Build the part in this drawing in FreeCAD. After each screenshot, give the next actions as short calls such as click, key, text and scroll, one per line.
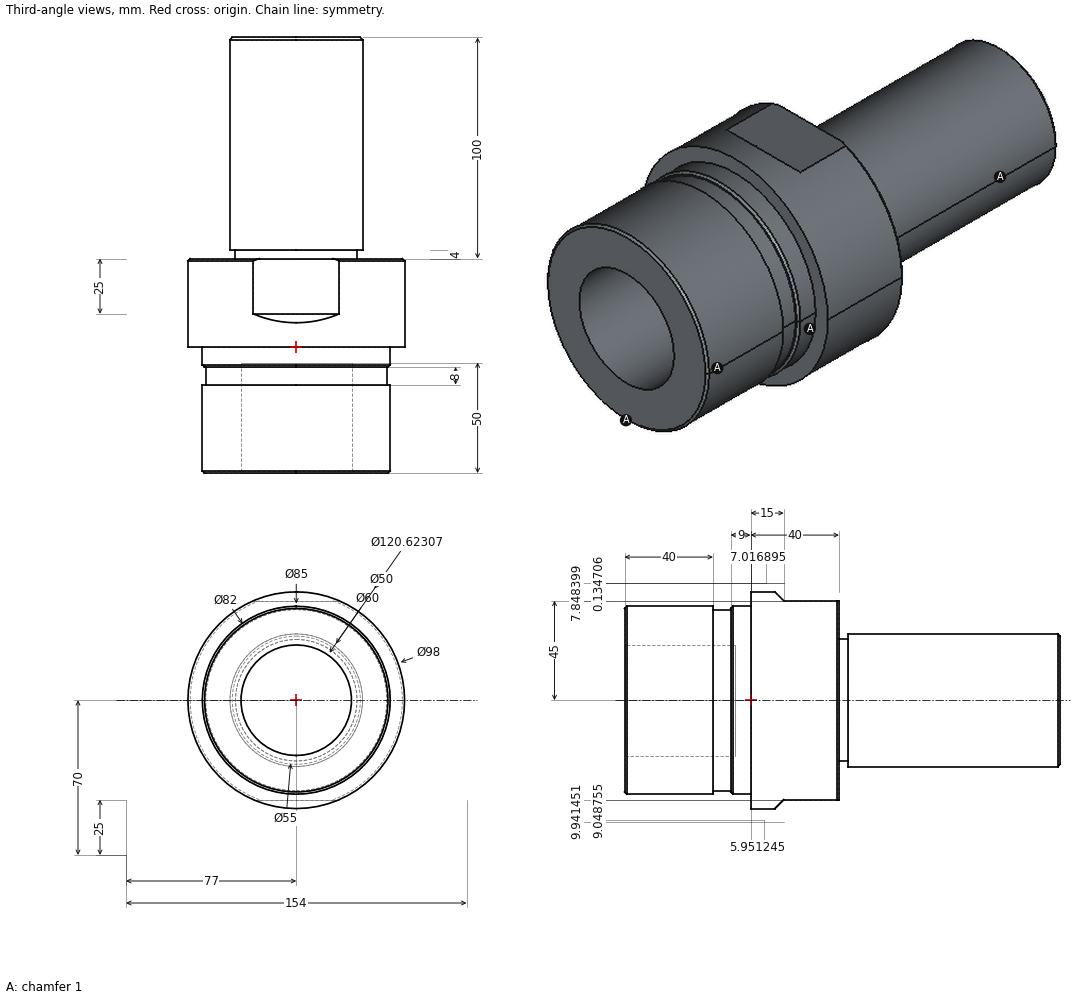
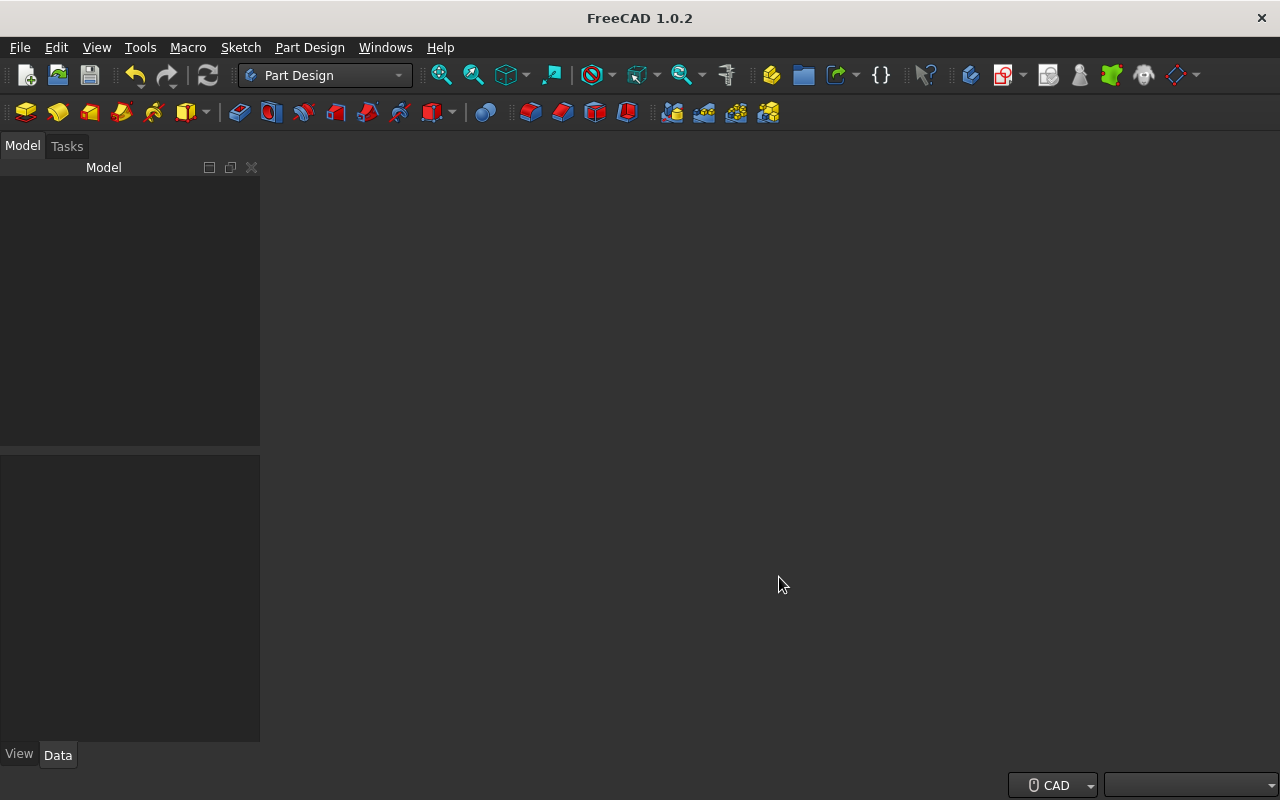
click(26, 76)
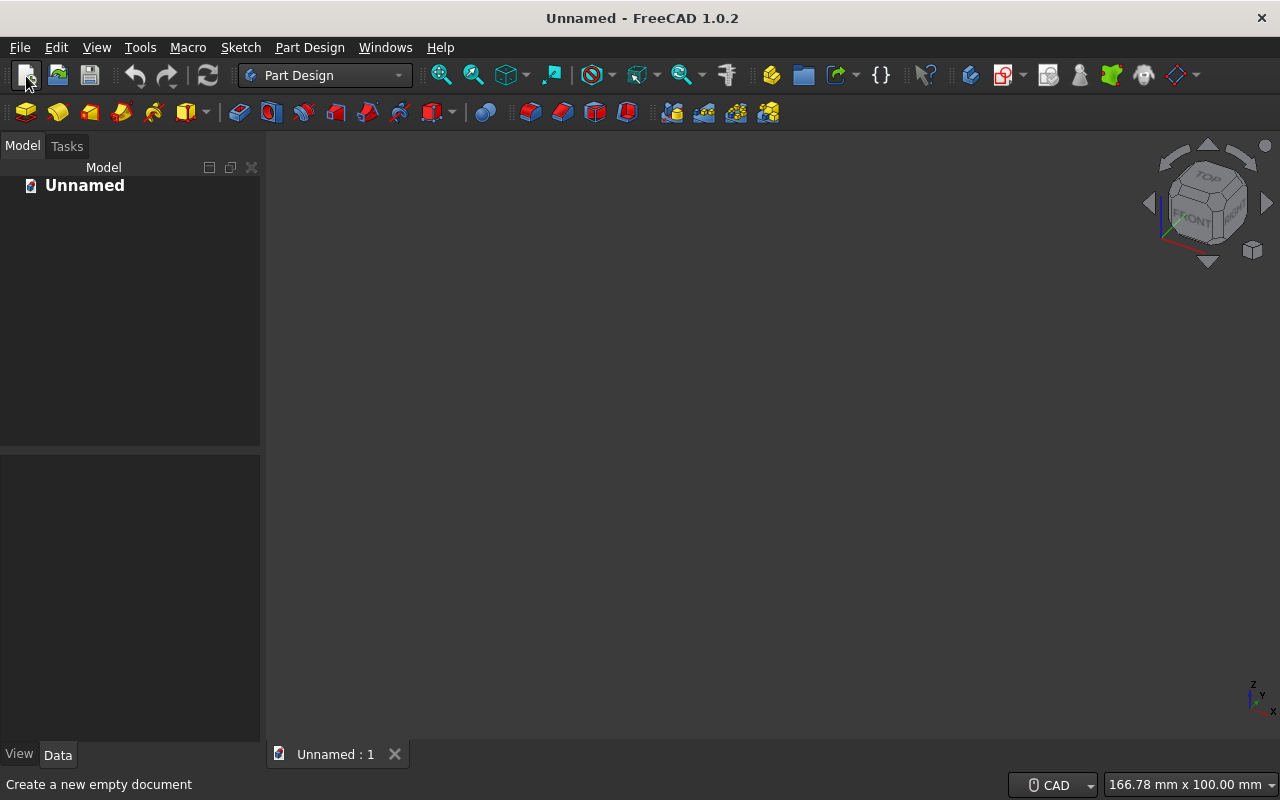
click(1004, 76)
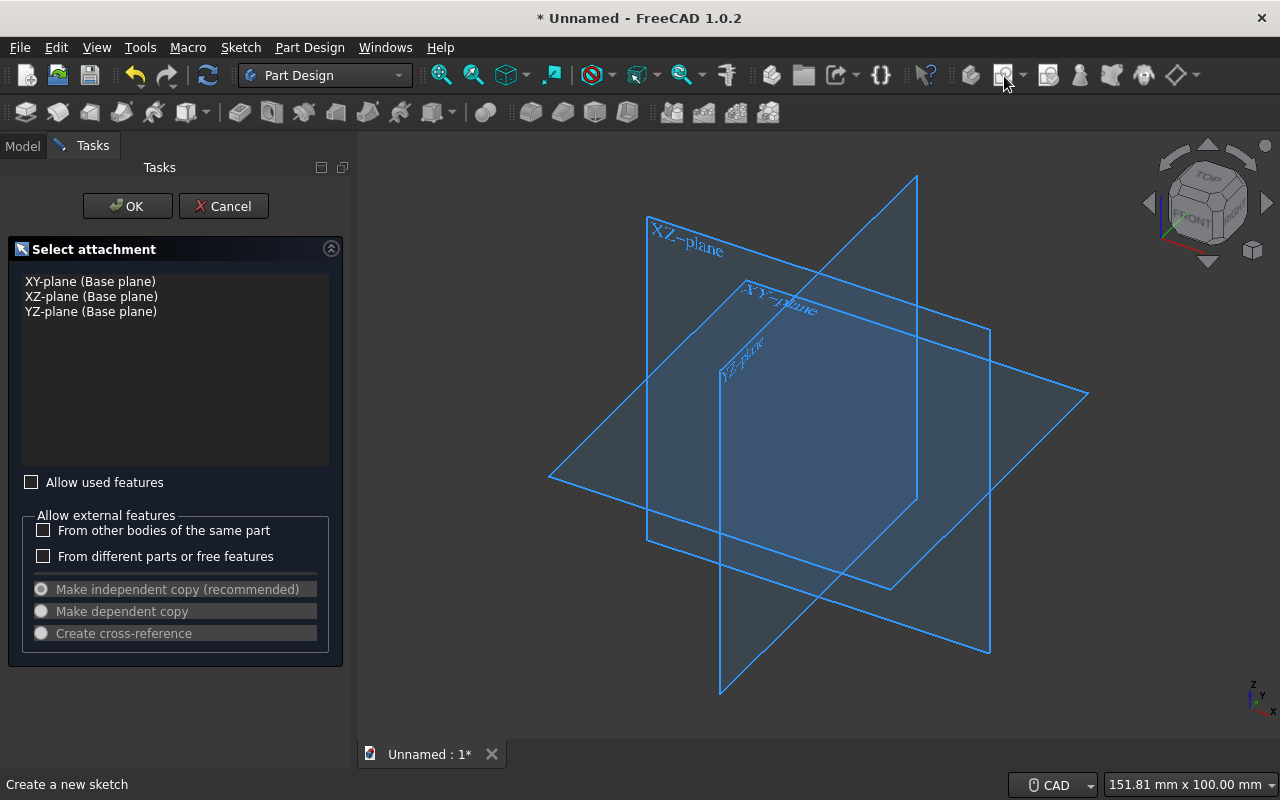
click(82, 296)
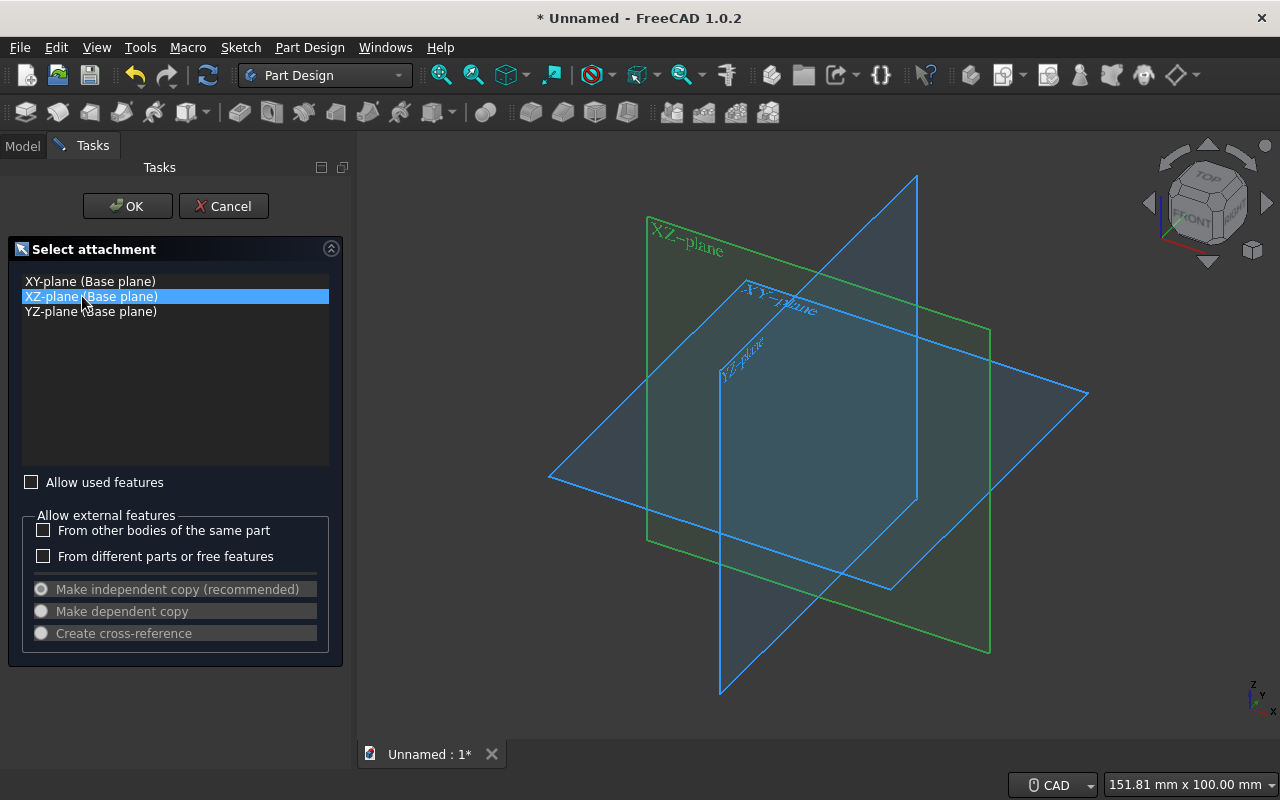
click(128, 206)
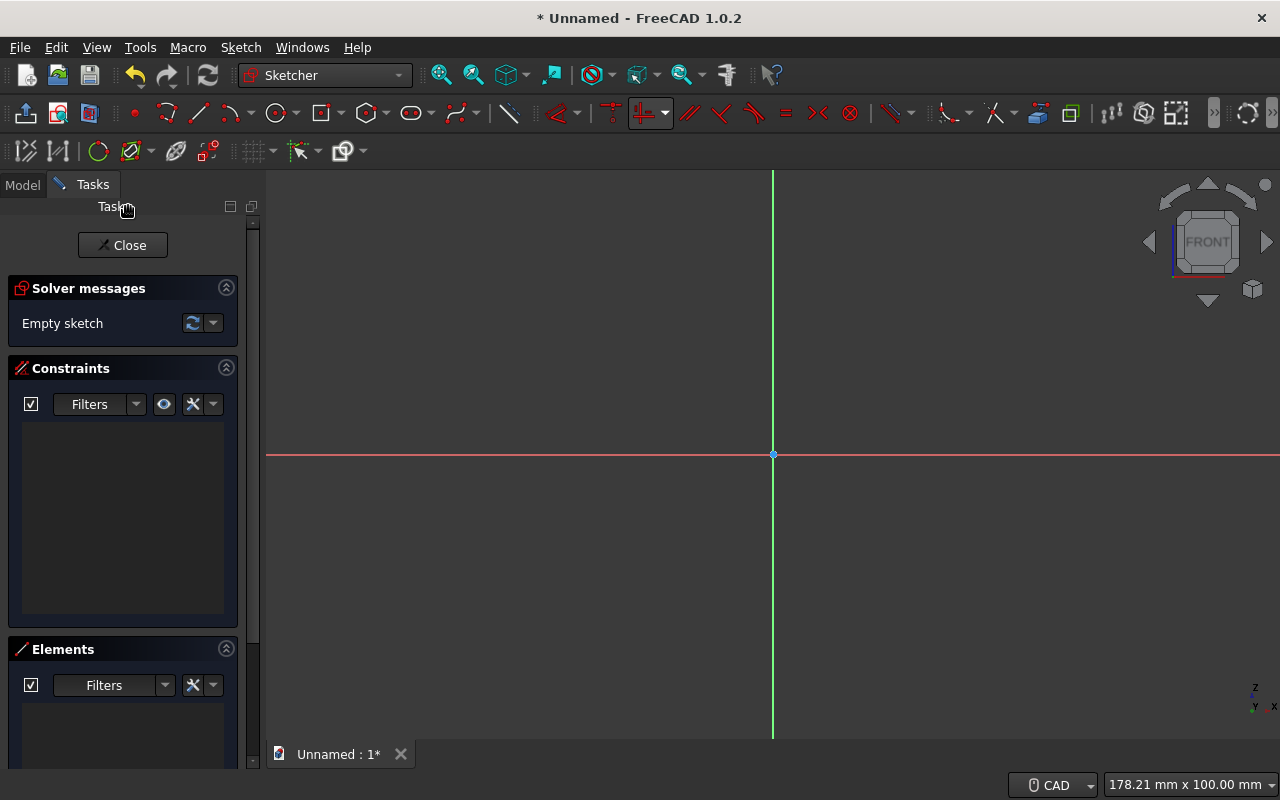
scroll(565, 455, down, 2)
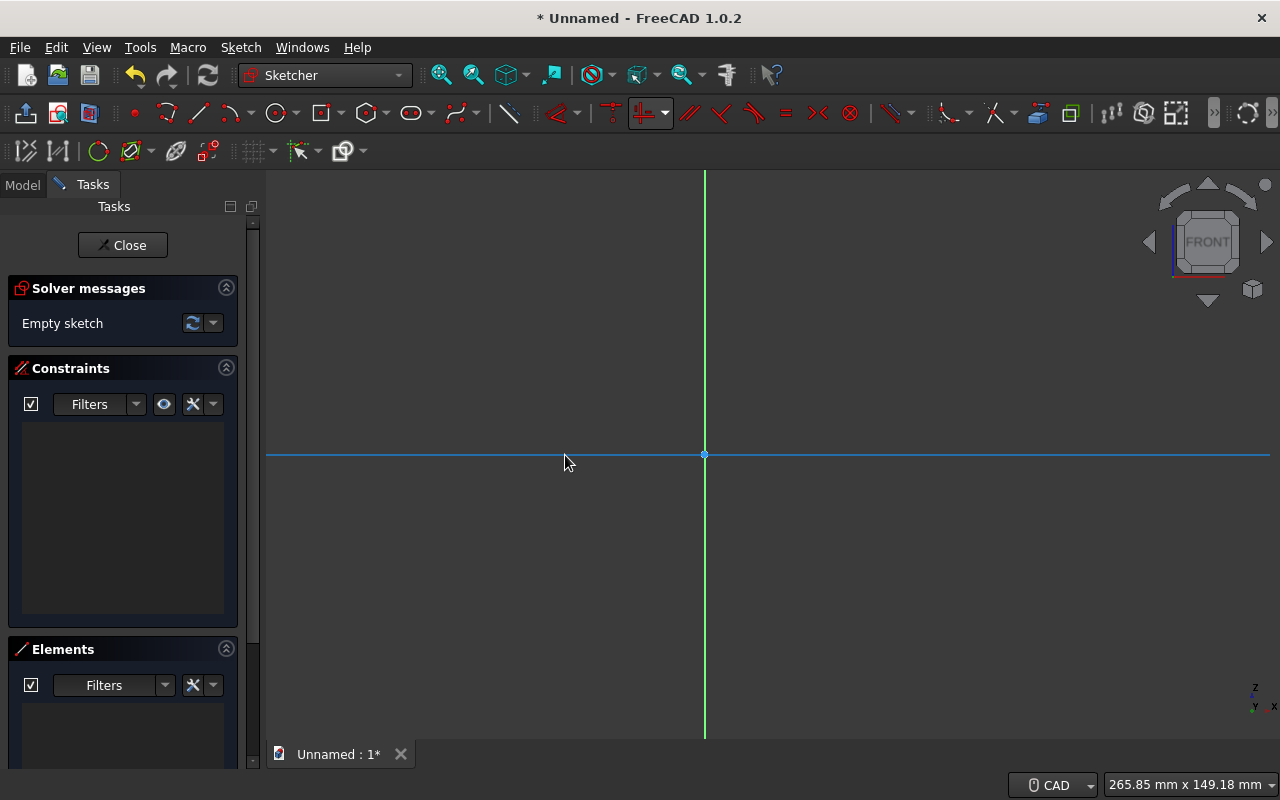
click(276, 114)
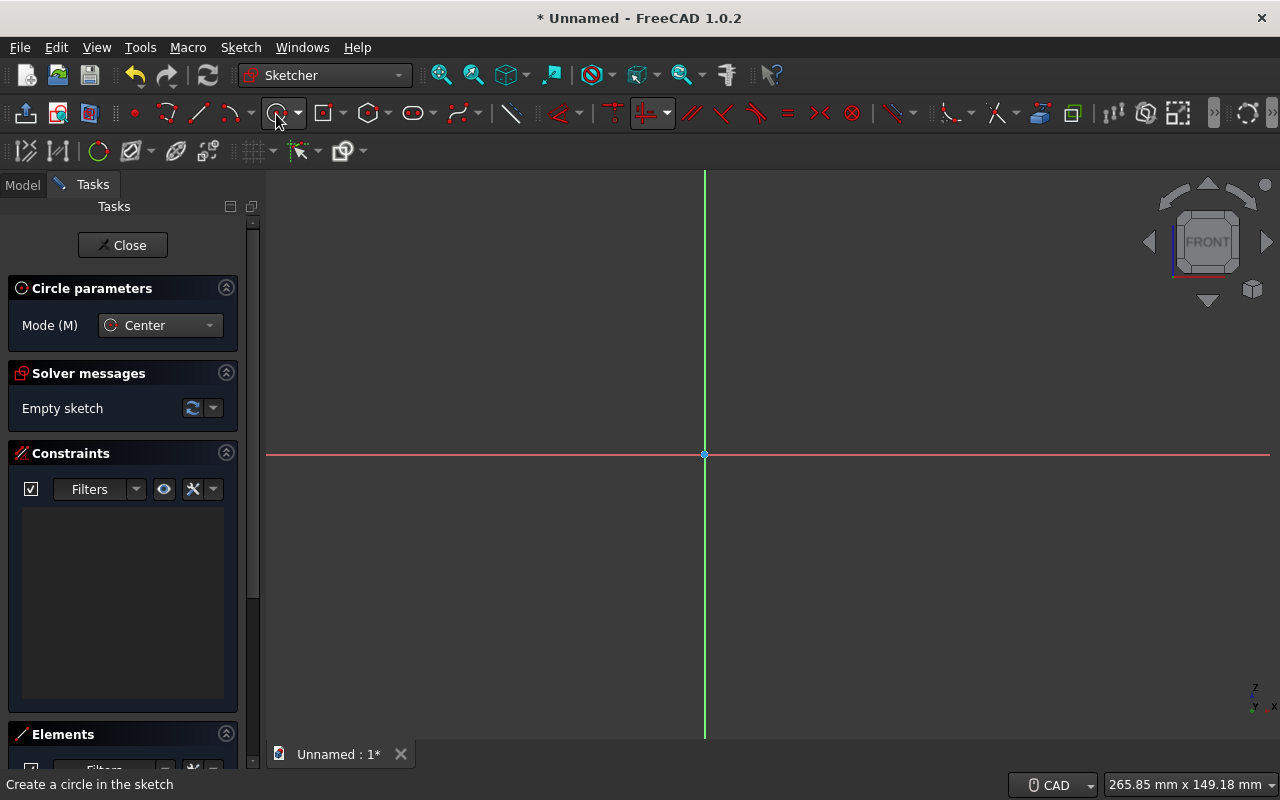
click(705, 455)
click(837, 323)
key(Escape)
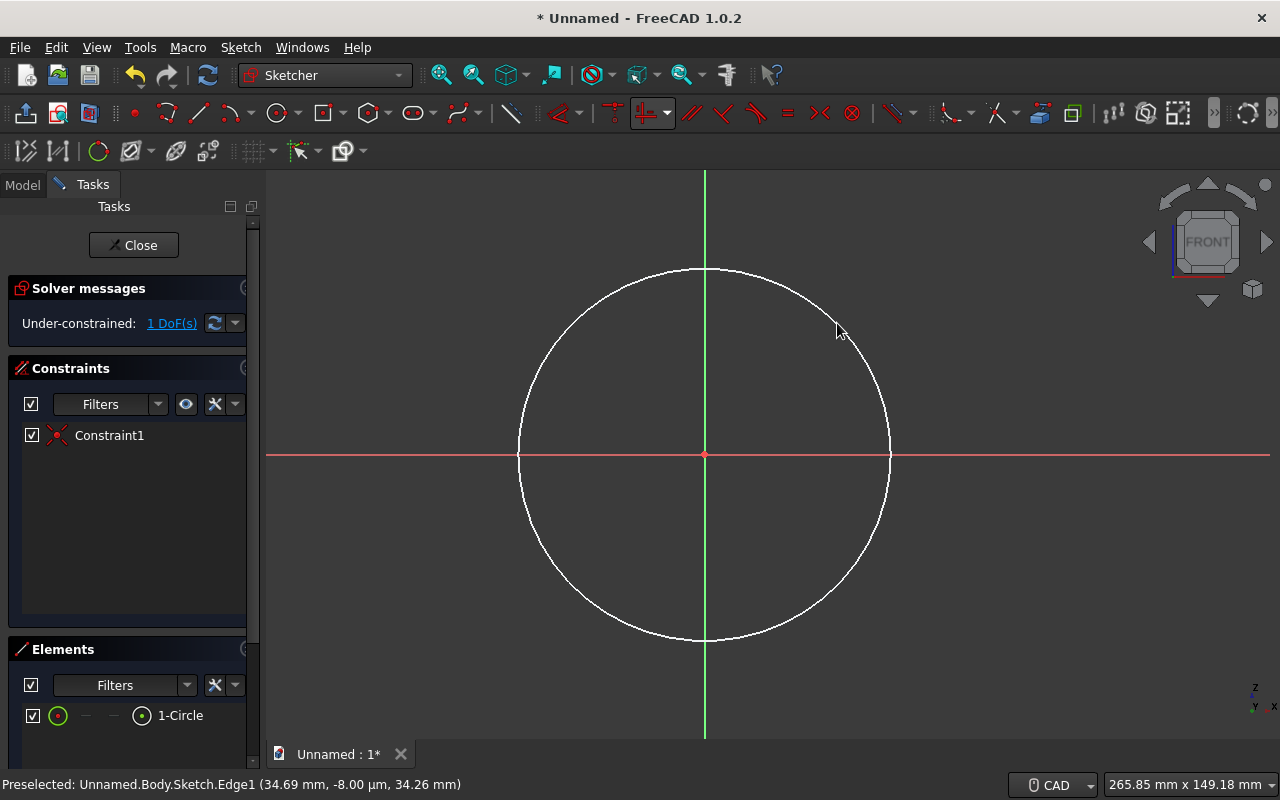
click(558, 114)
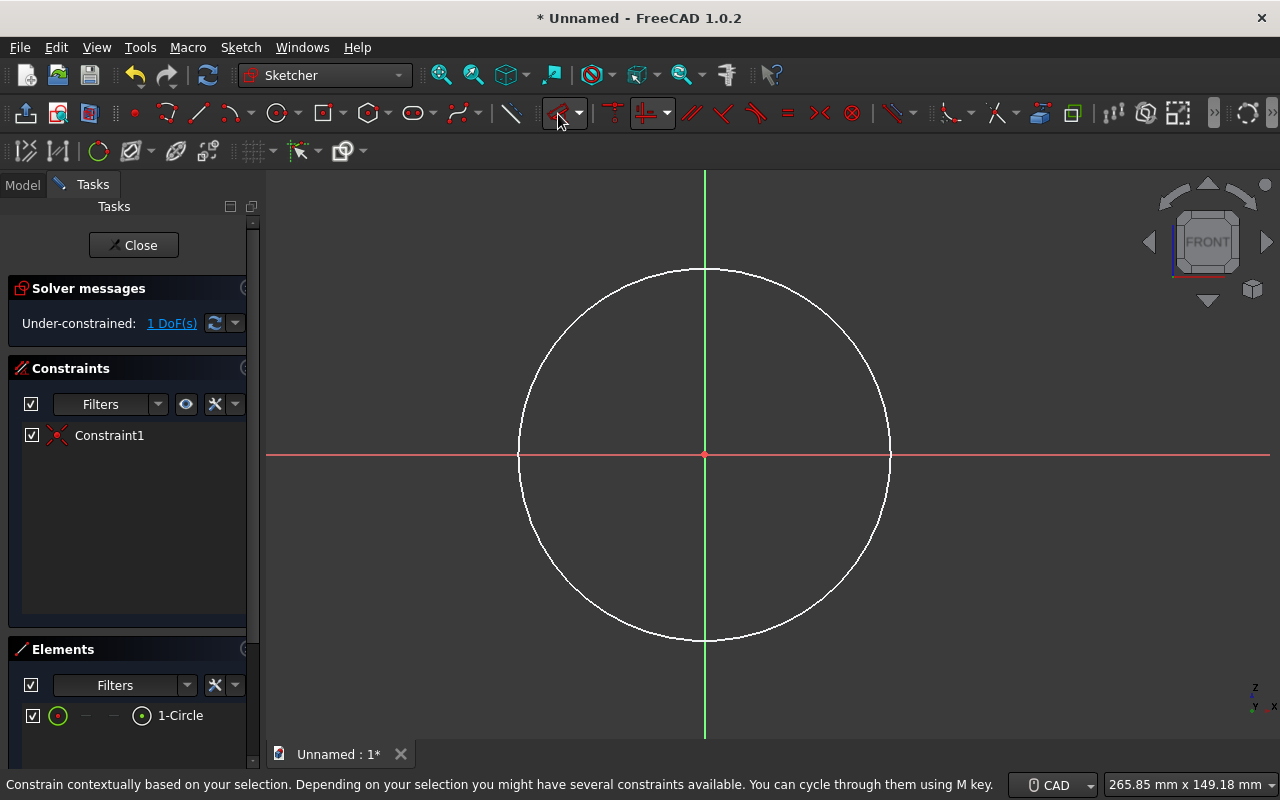
click(836, 323)
click(859, 300)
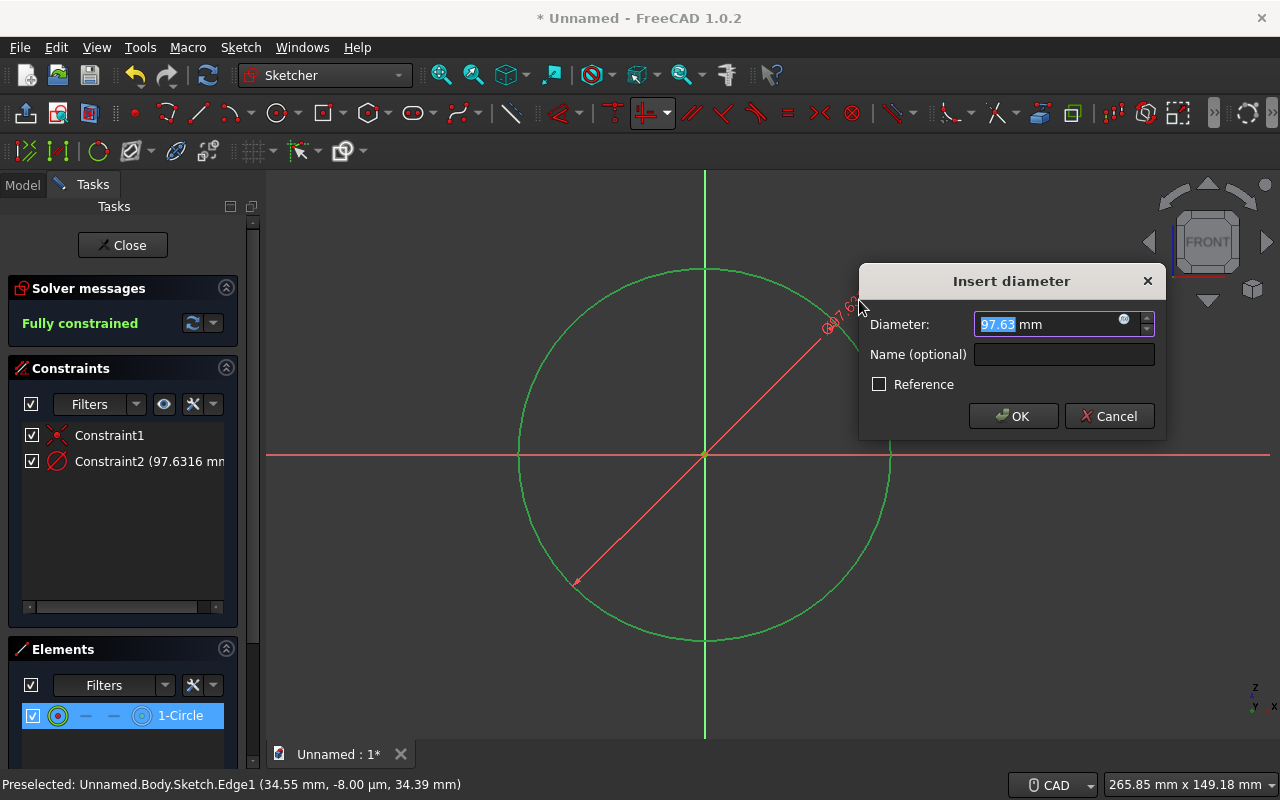
text(98)
key(Return)
key(Escape)